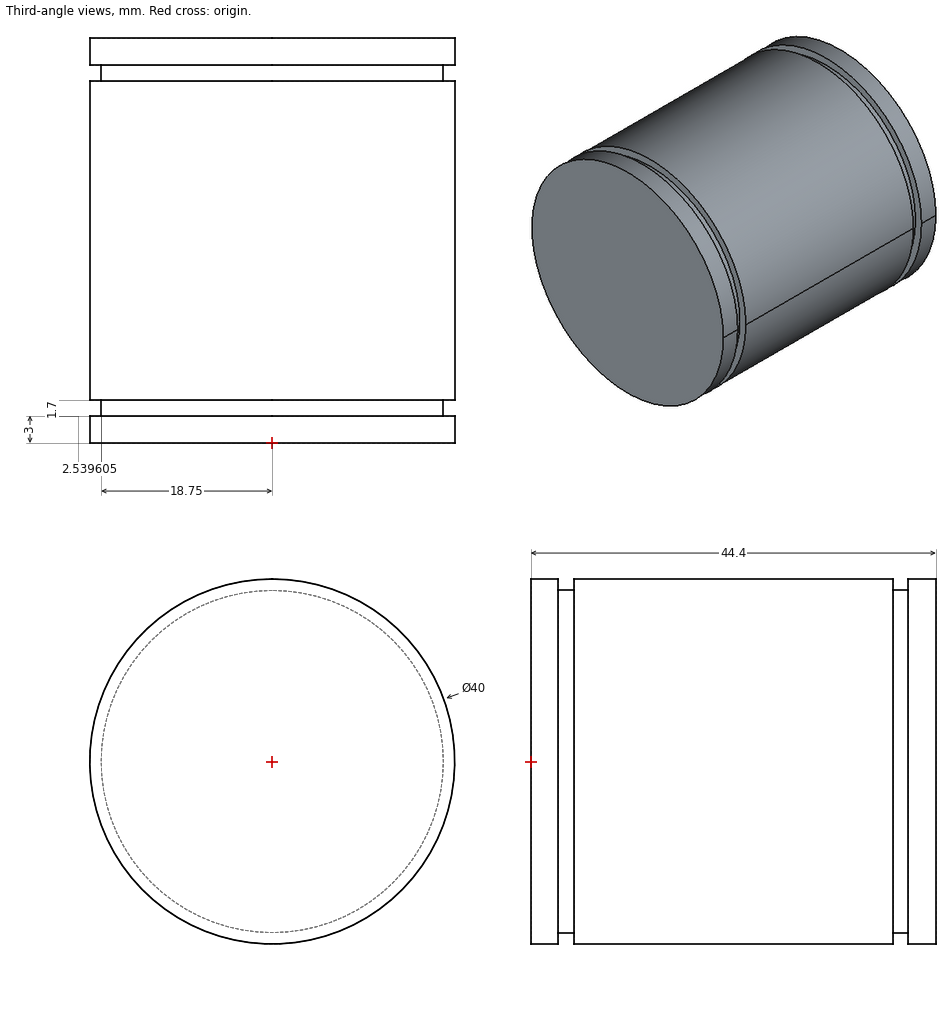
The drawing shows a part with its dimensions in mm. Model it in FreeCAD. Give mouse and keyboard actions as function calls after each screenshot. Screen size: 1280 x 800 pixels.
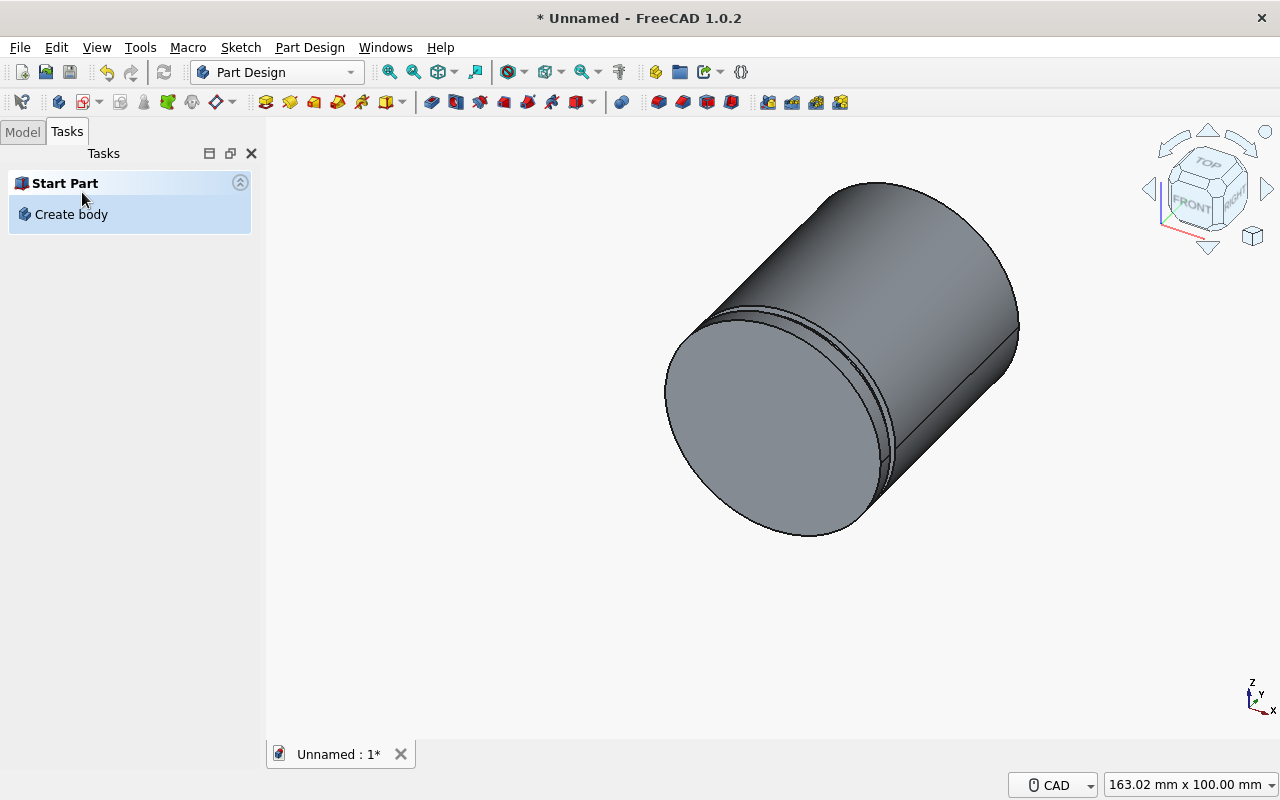
click(23, 131)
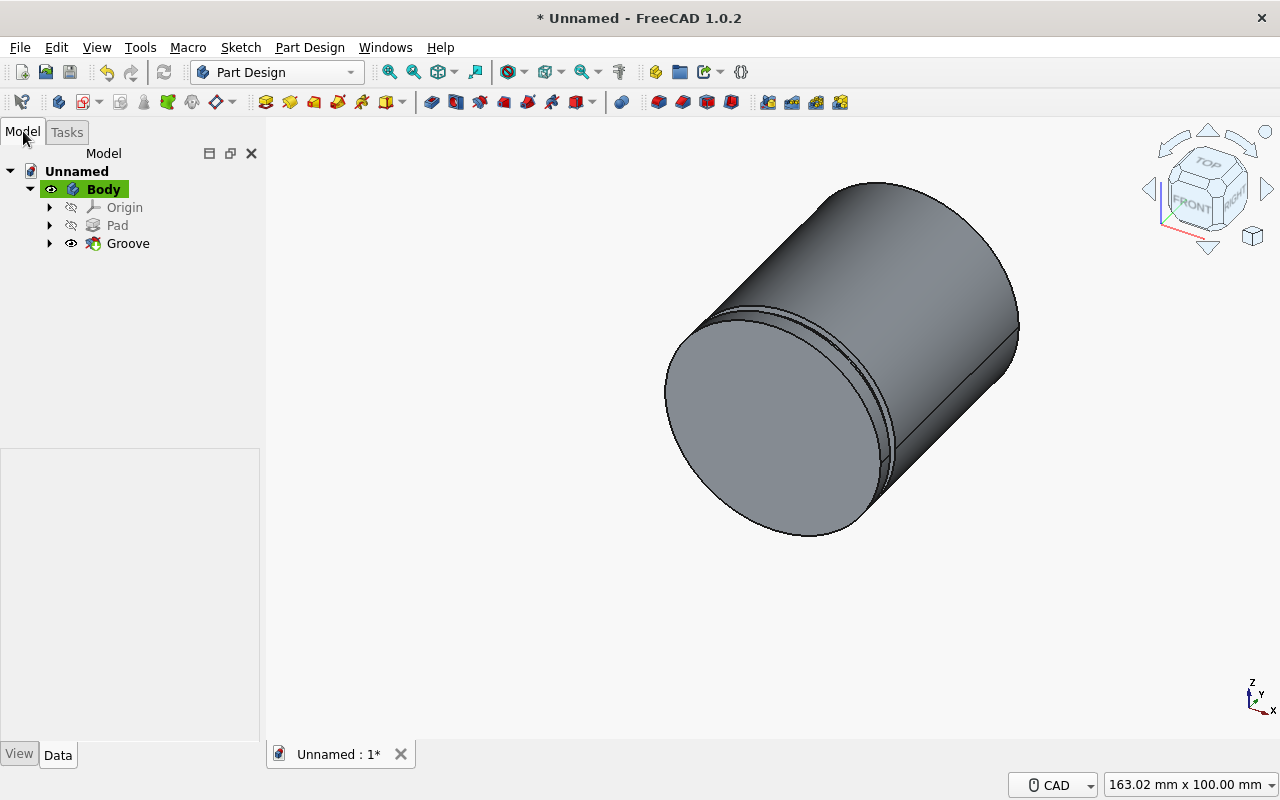
click(50, 207)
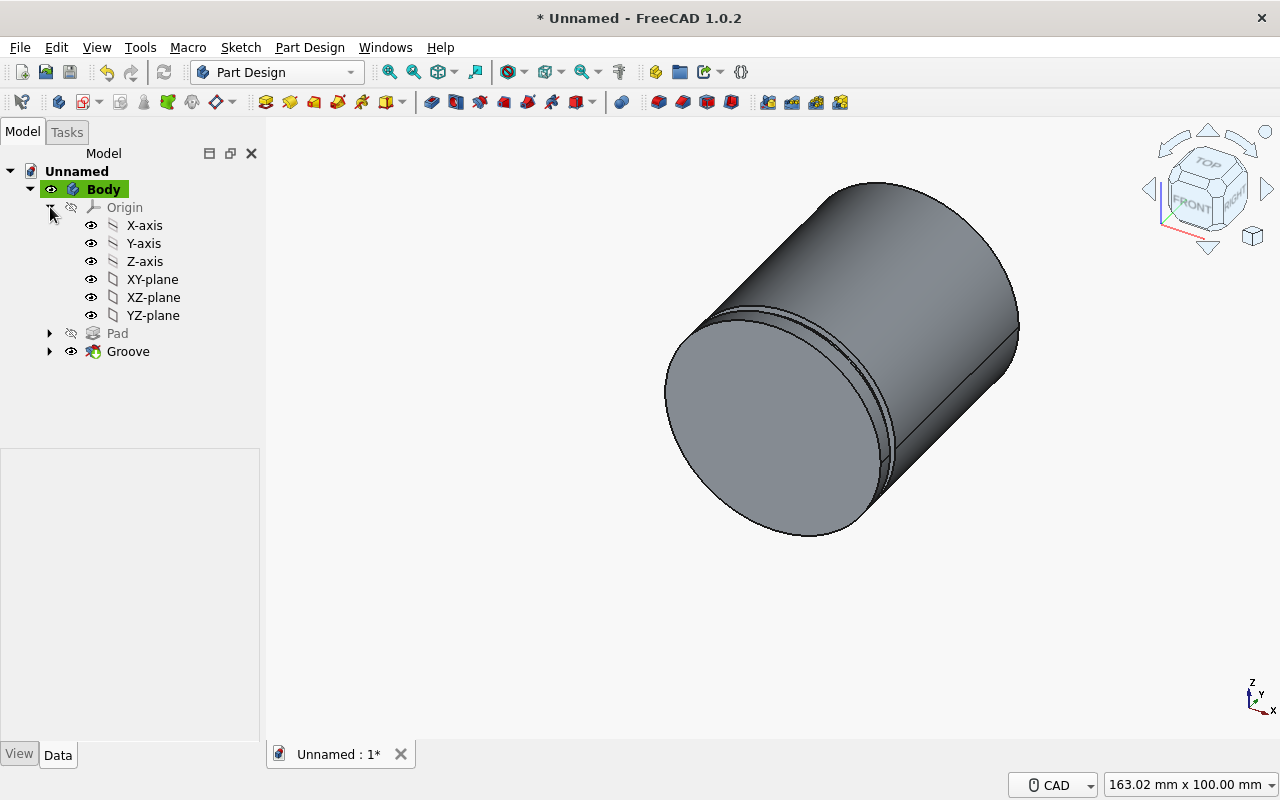
click(136, 297)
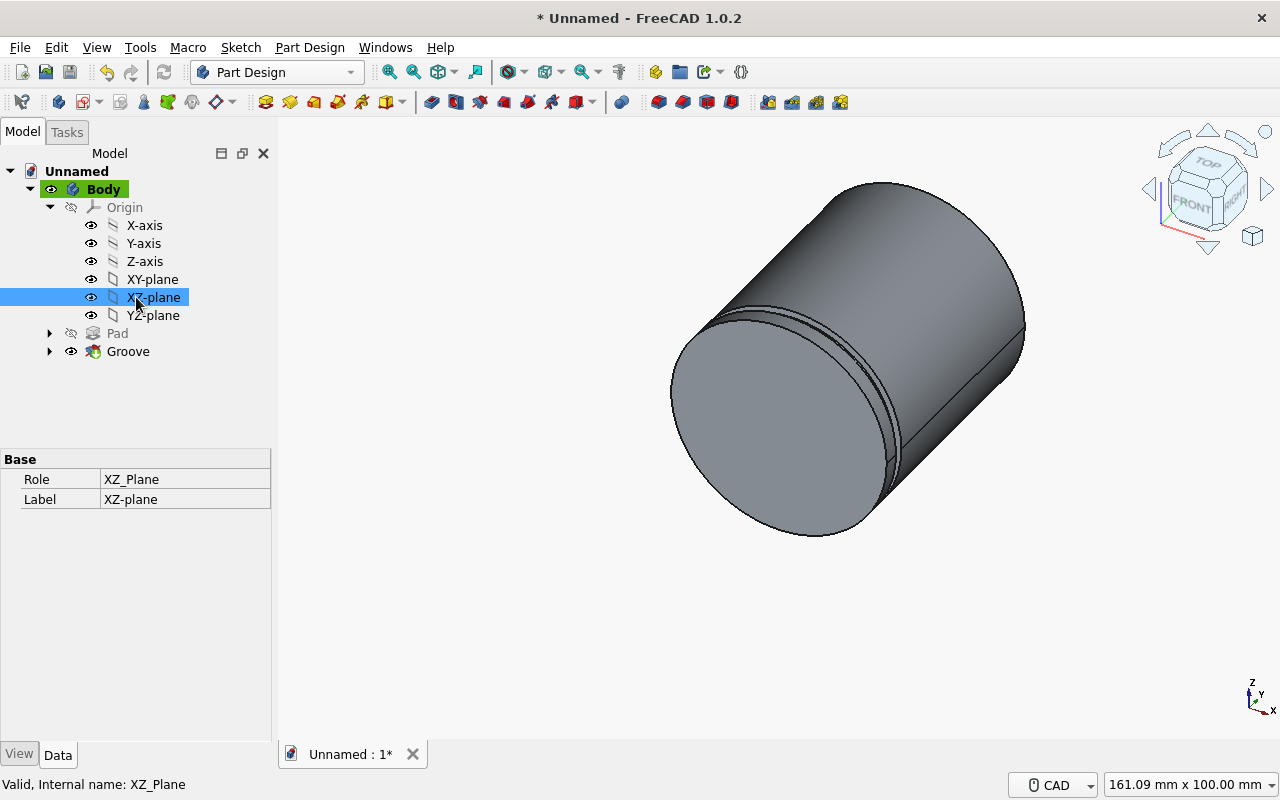
click(216, 102)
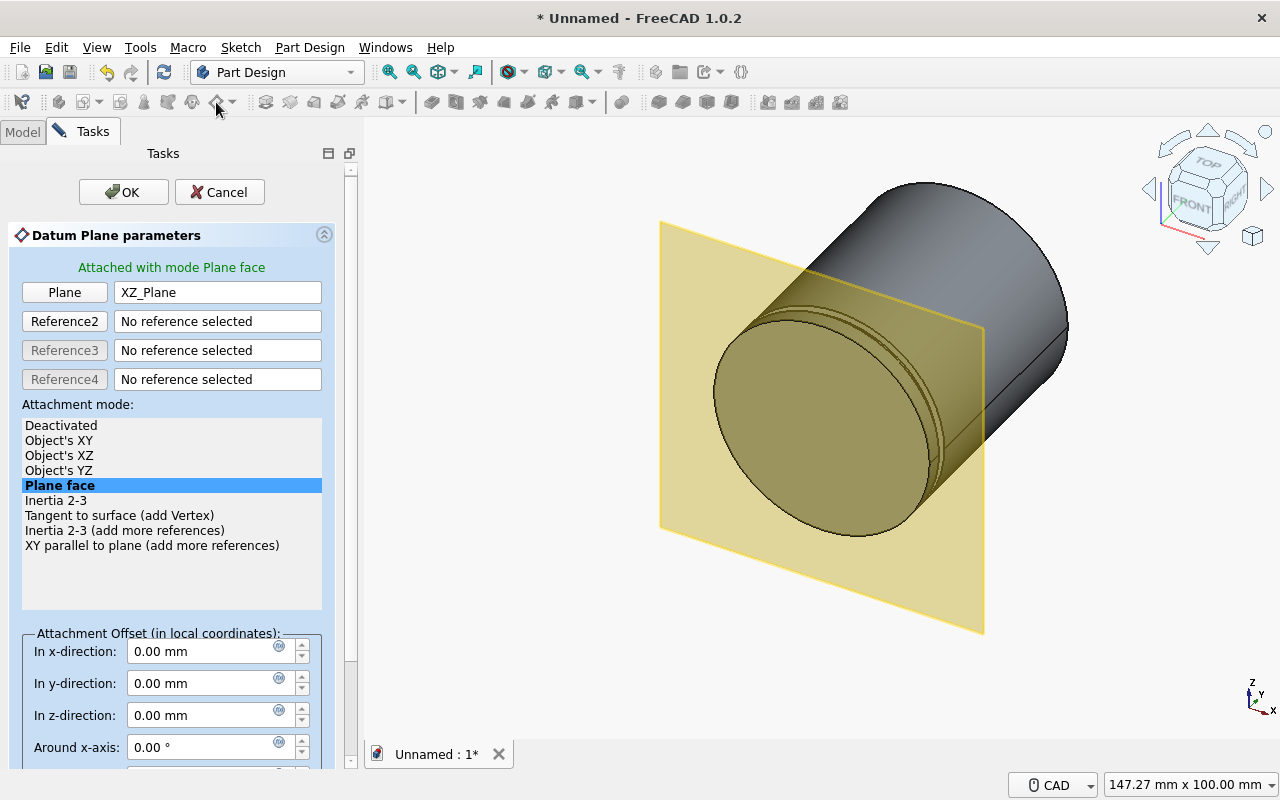
triple_click(210, 715)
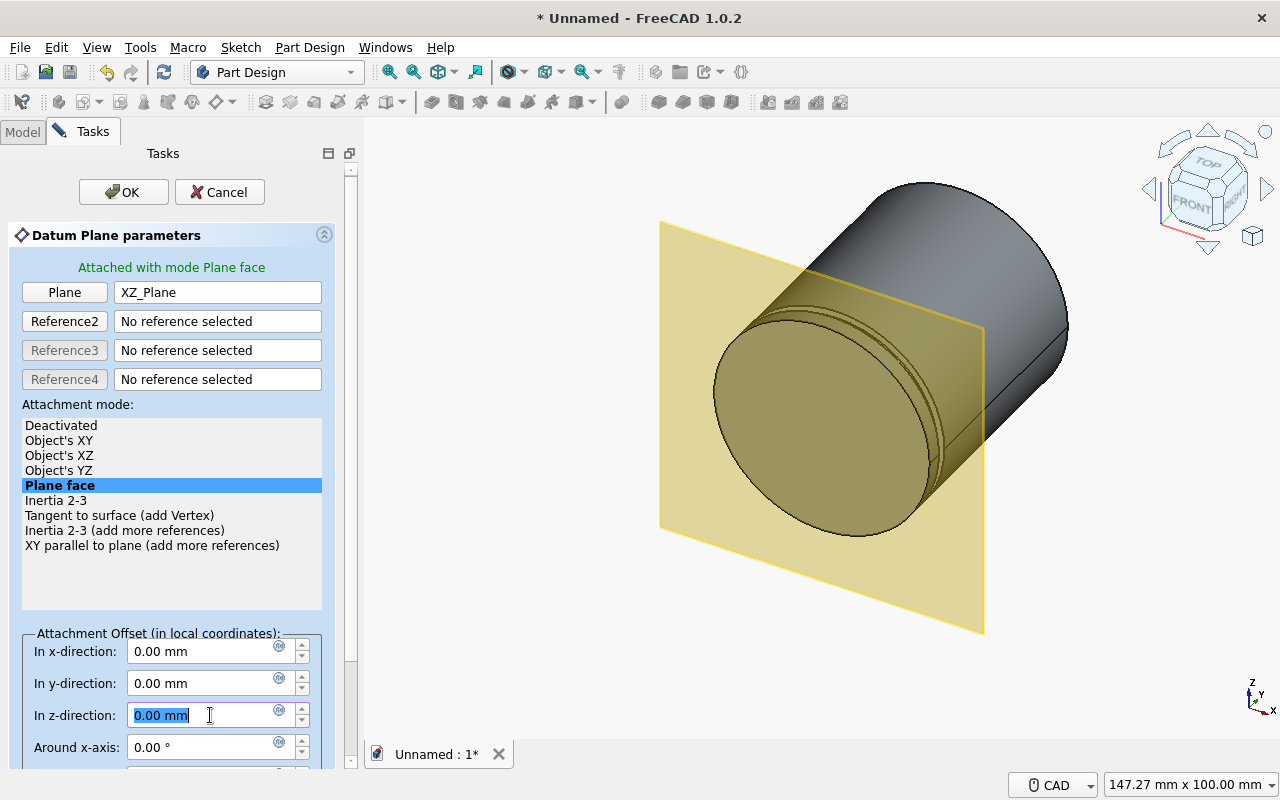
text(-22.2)
key(Tab)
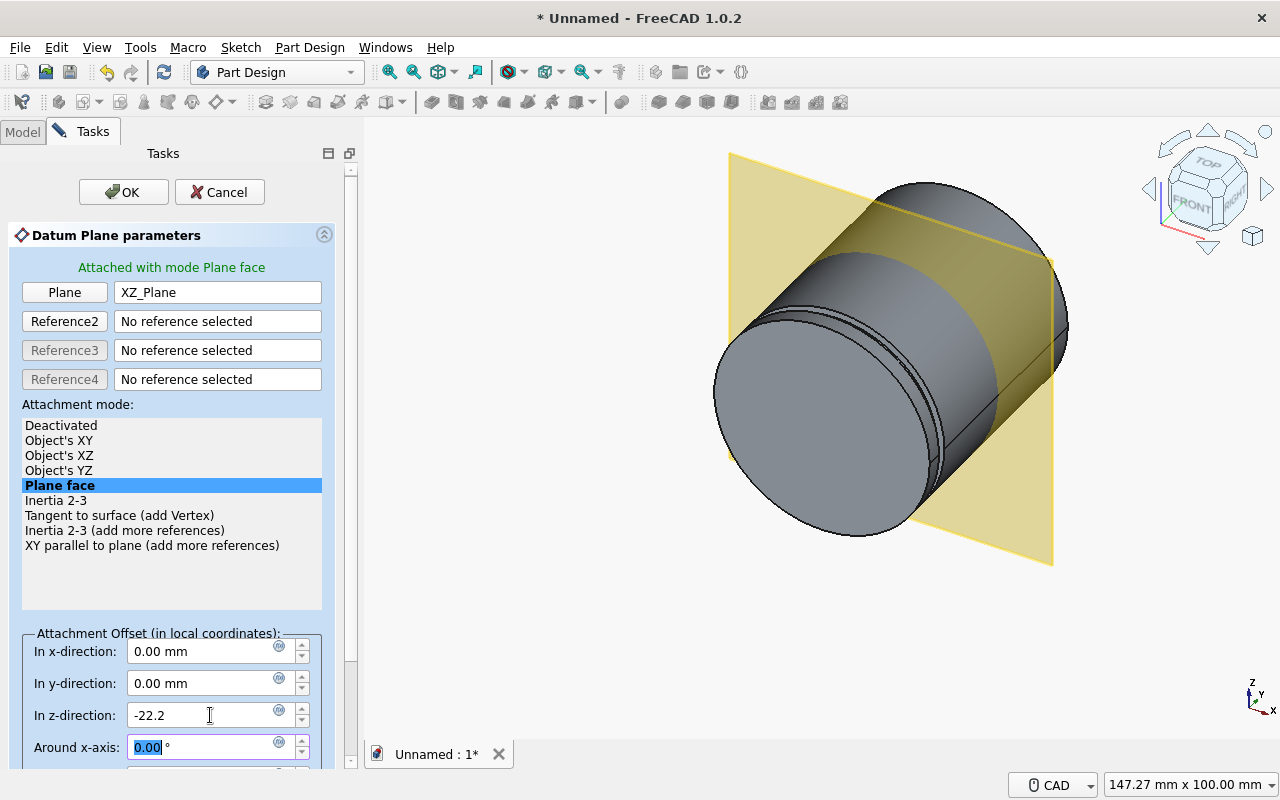
click(124, 192)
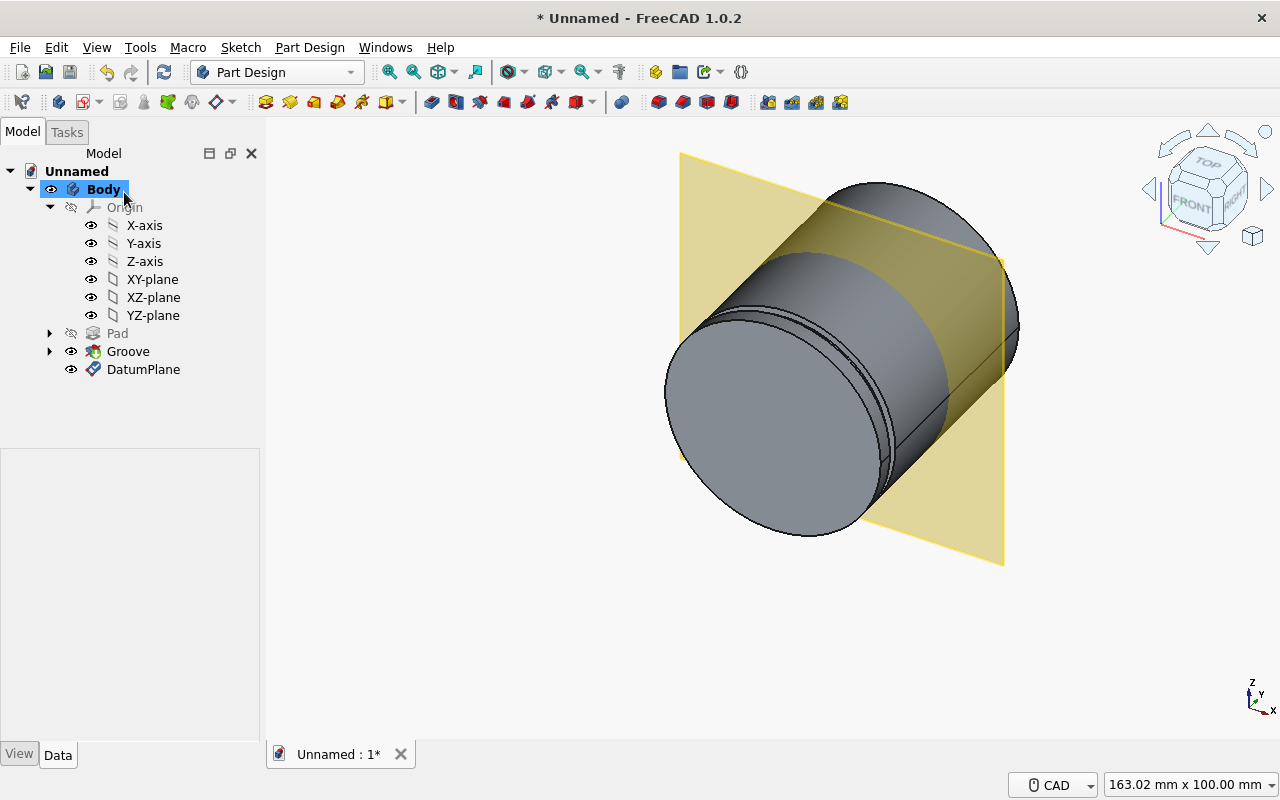
click(116, 351)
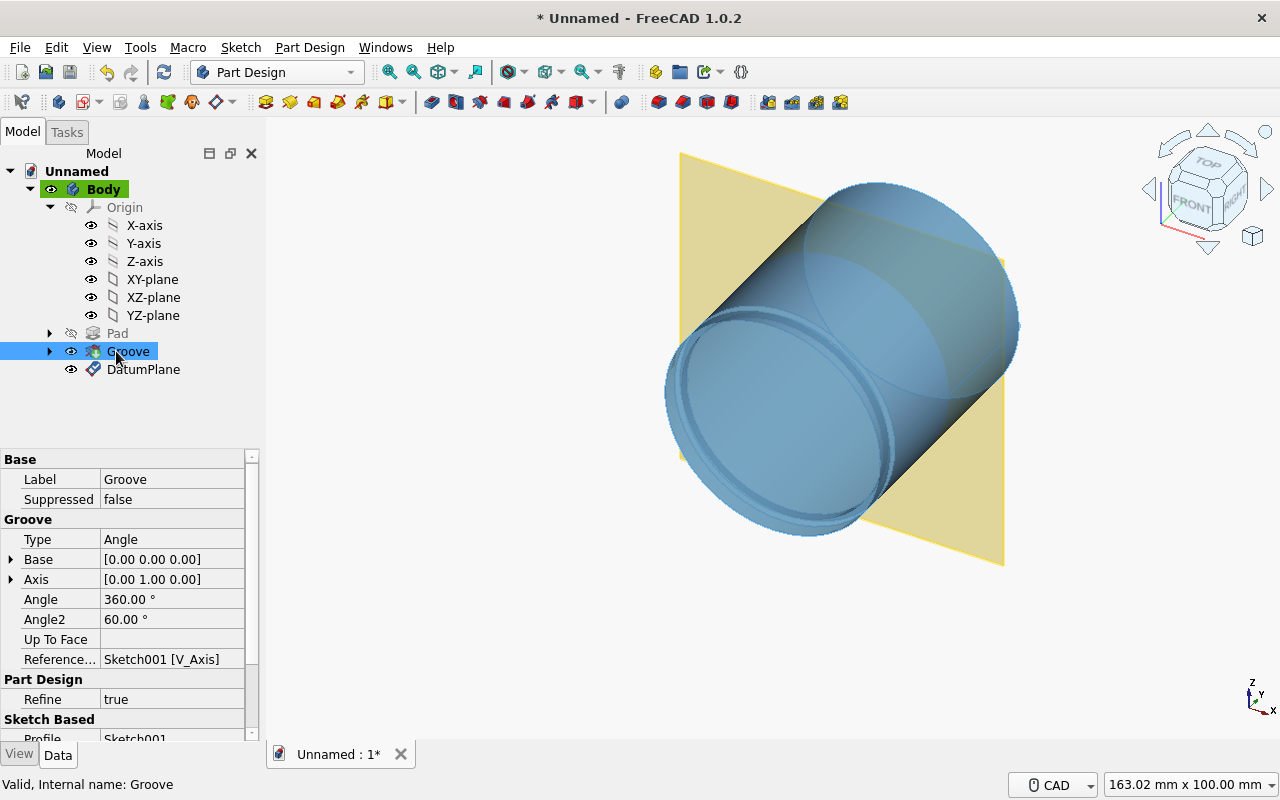
click(768, 102)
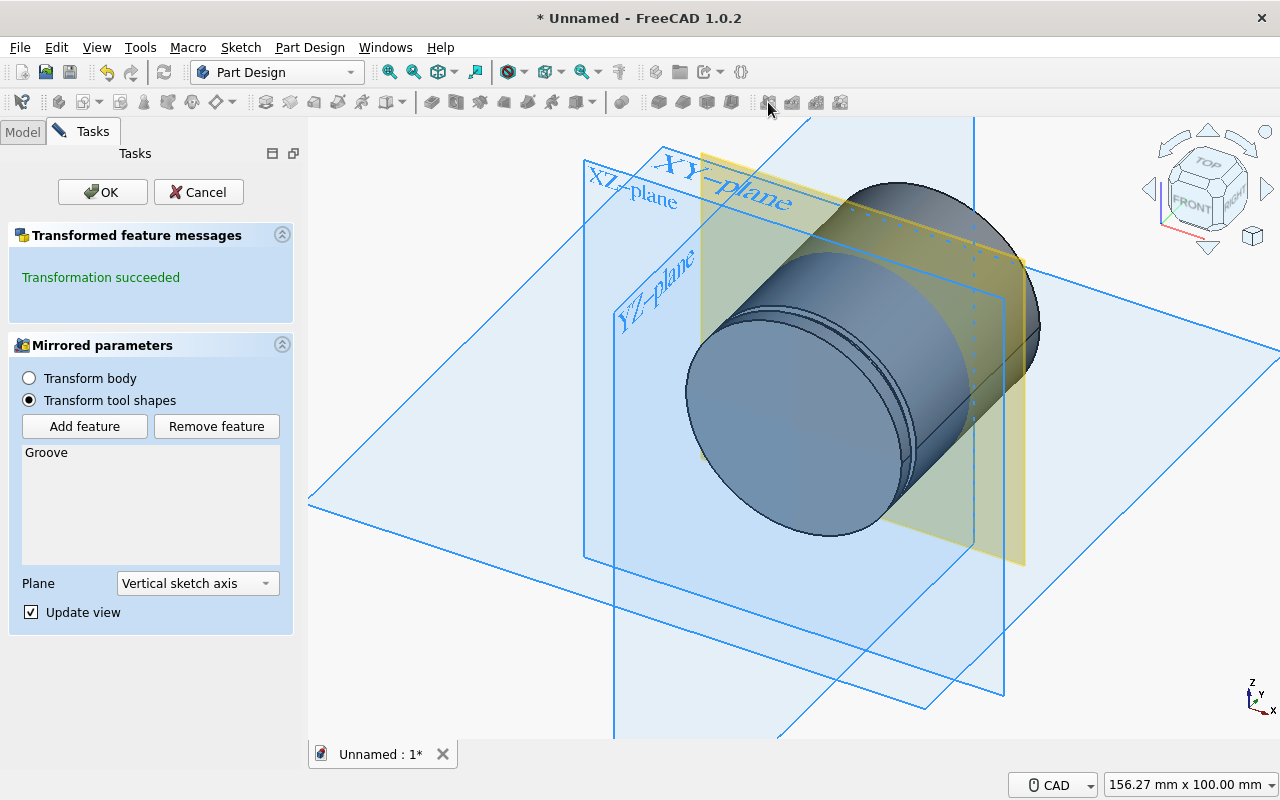
click(198, 584)